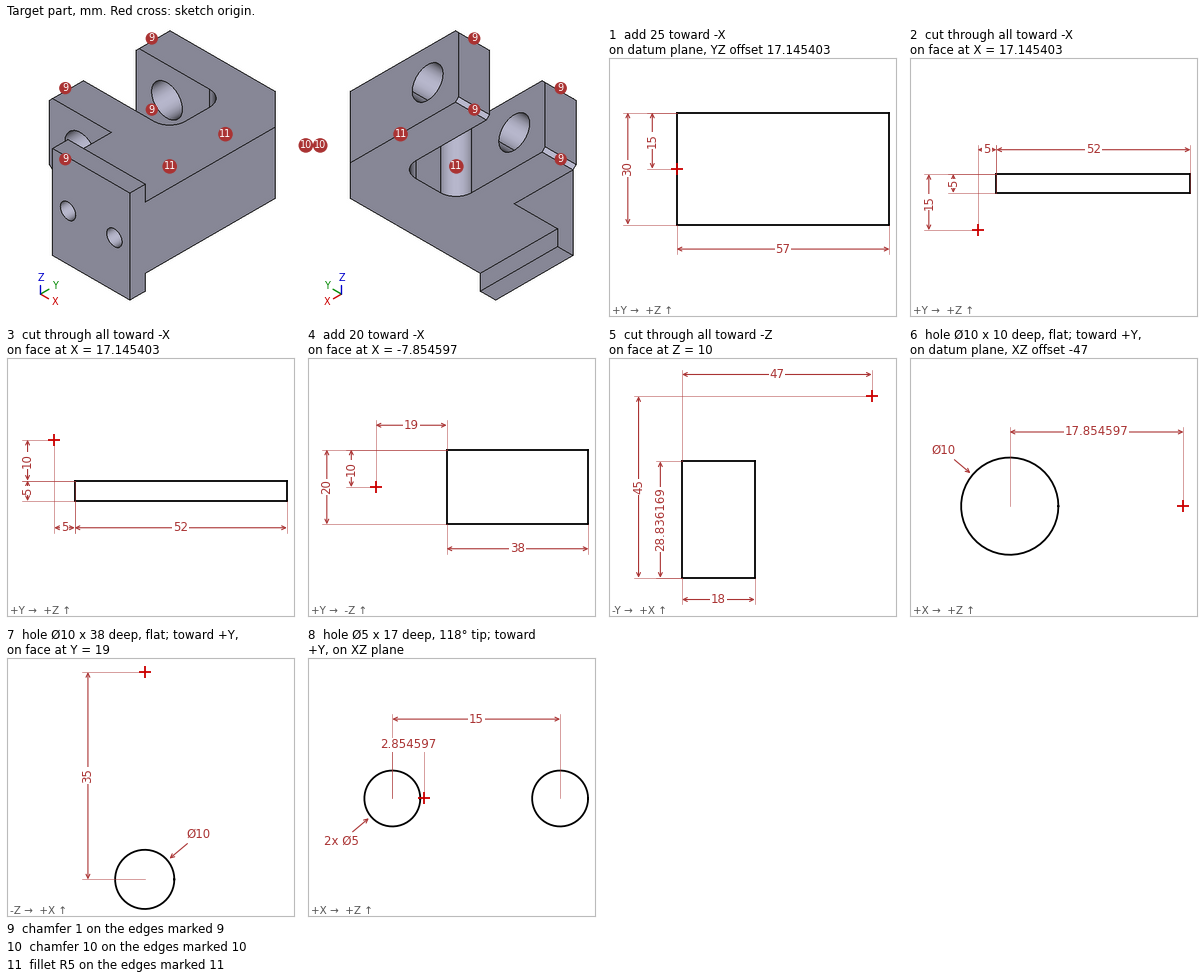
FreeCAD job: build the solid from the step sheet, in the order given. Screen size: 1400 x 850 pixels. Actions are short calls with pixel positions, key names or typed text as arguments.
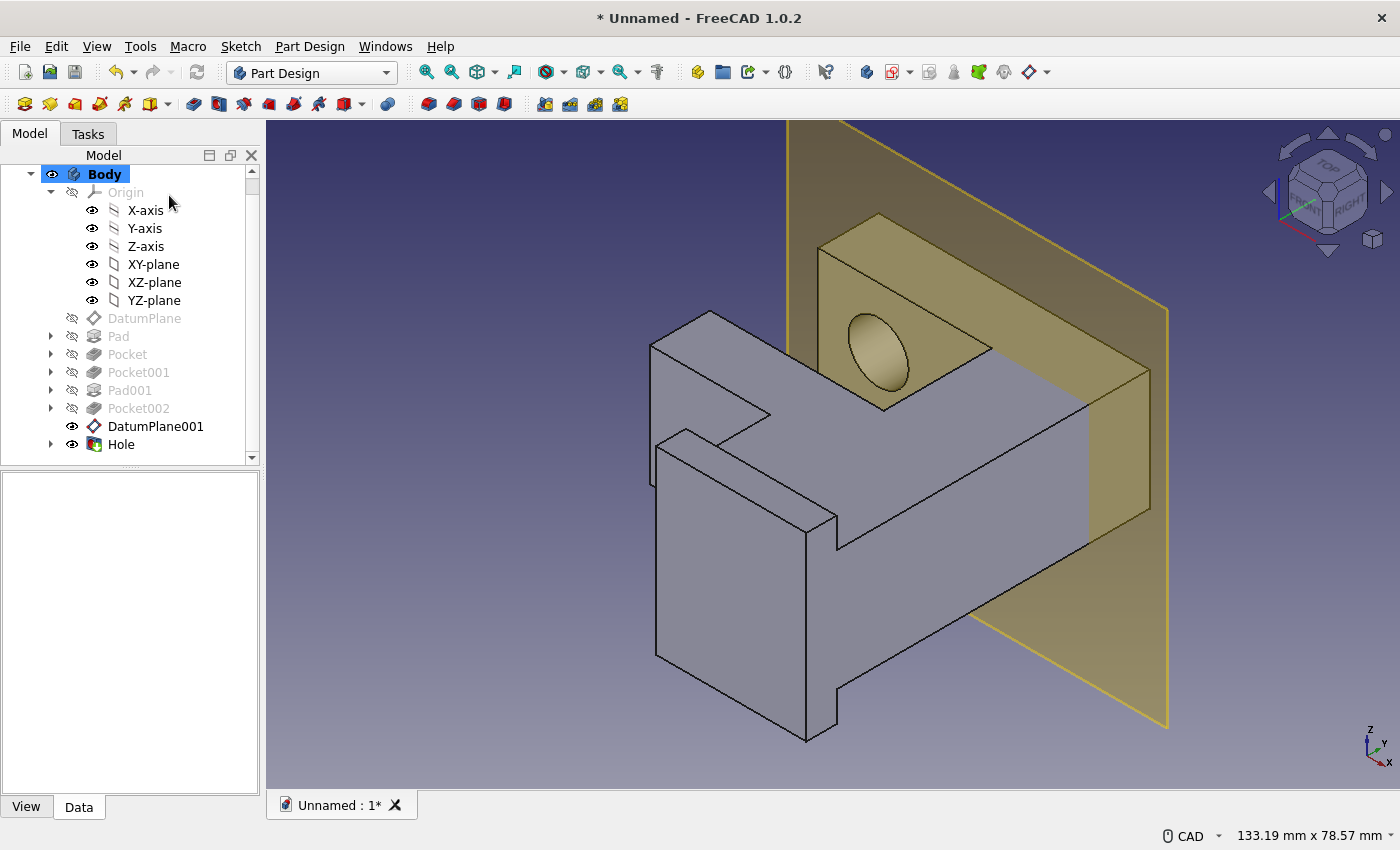
click(117, 426)
key(space)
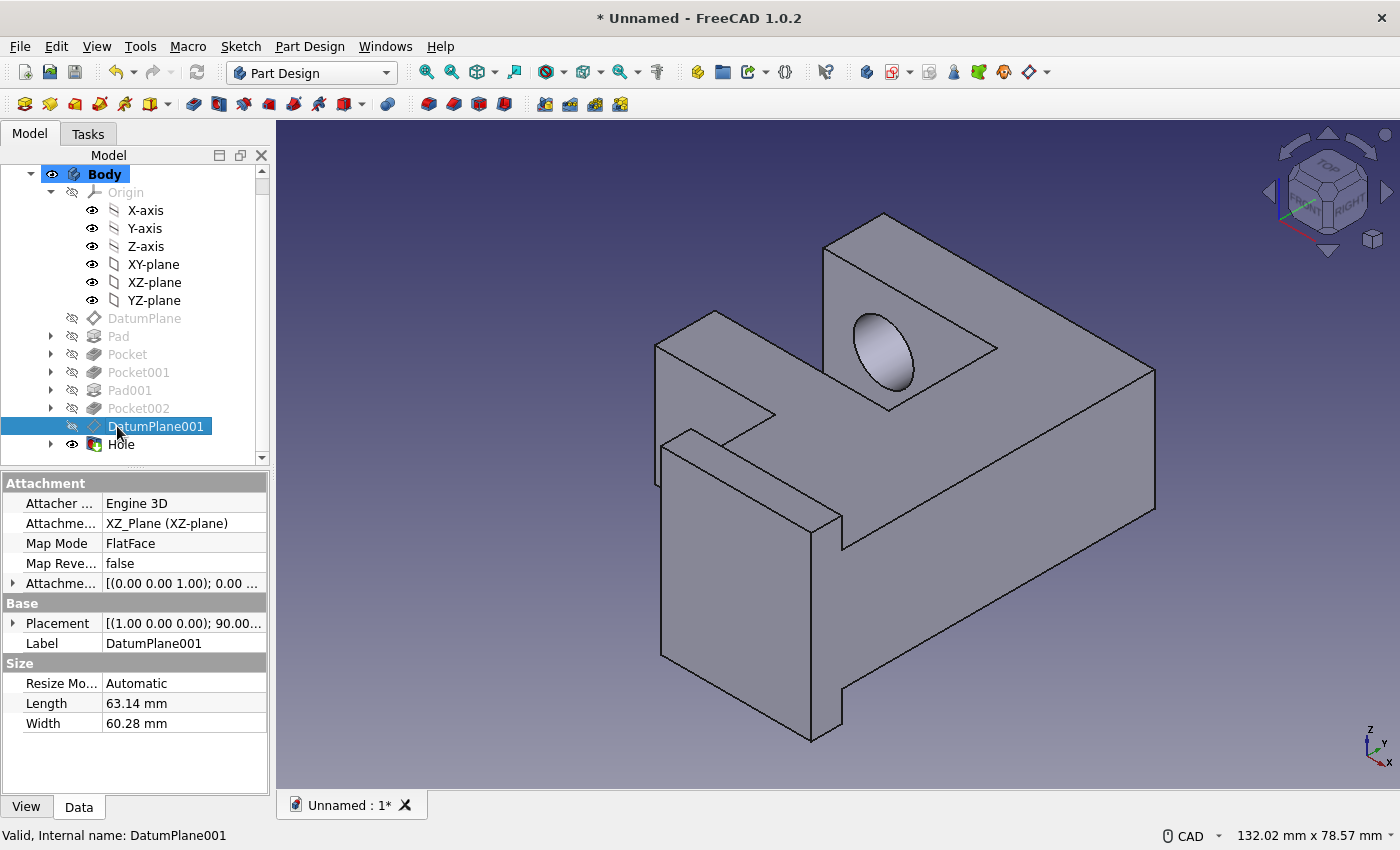
click(698, 419)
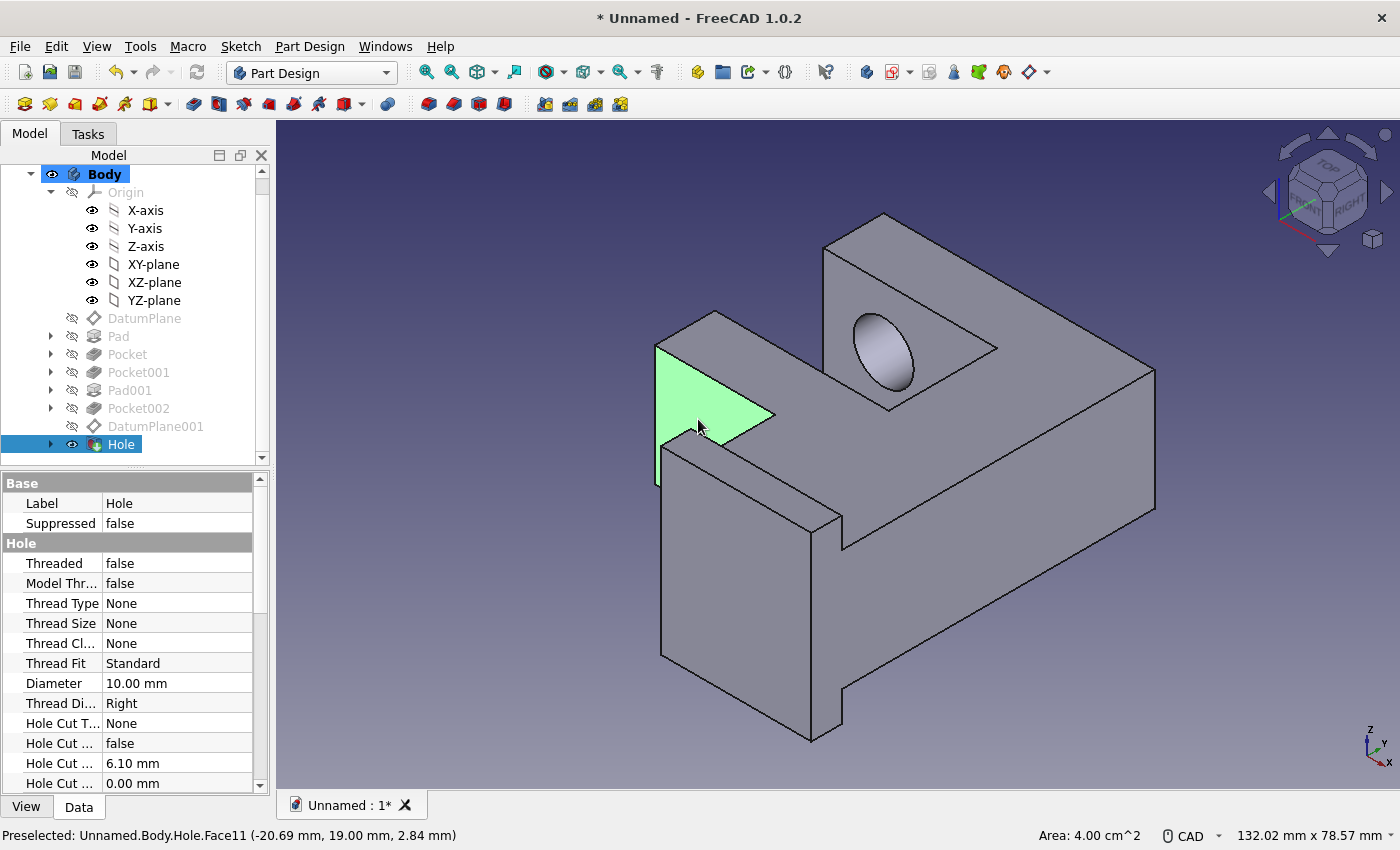
click(892, 72)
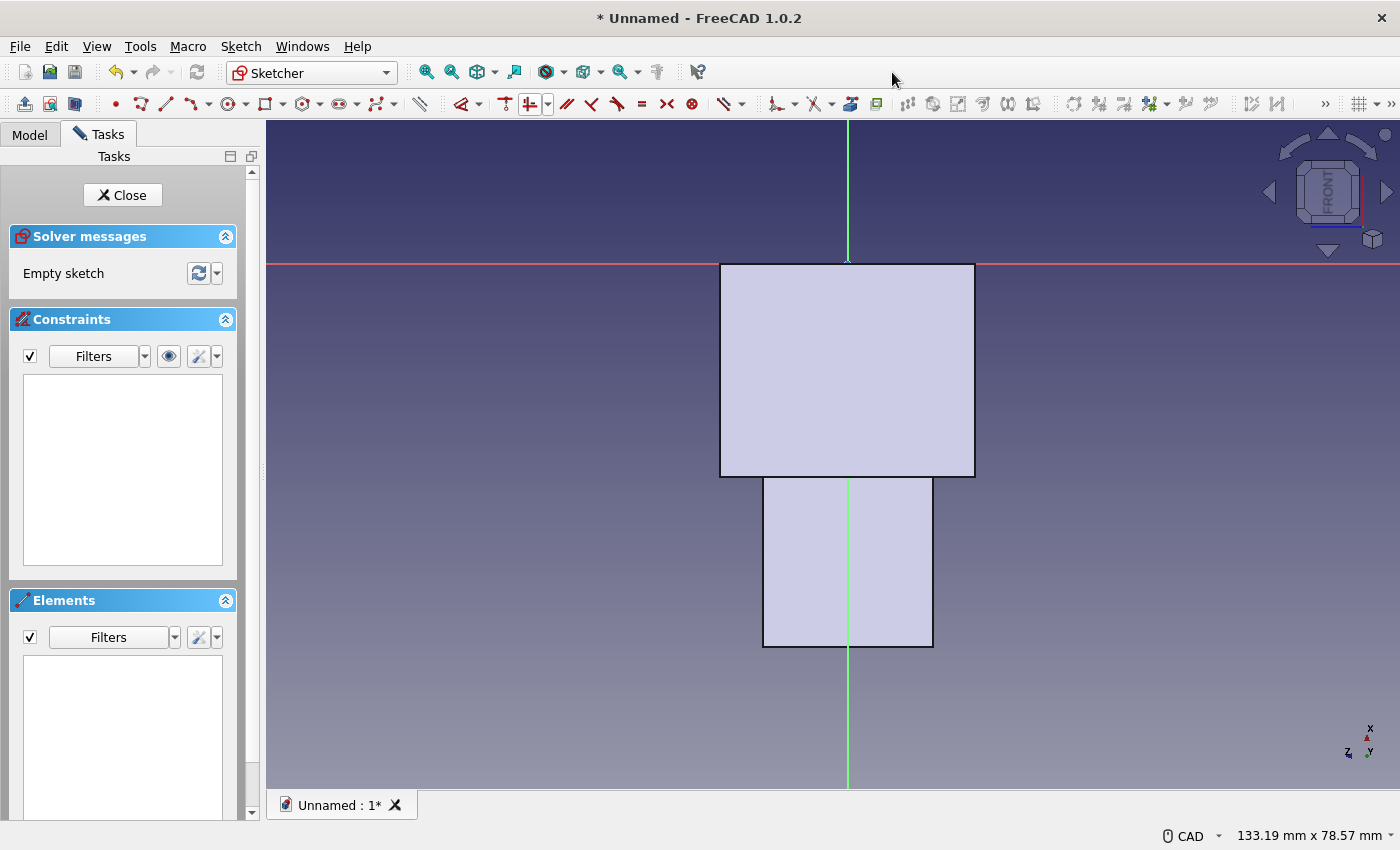
scroll(869, 589, up, 8)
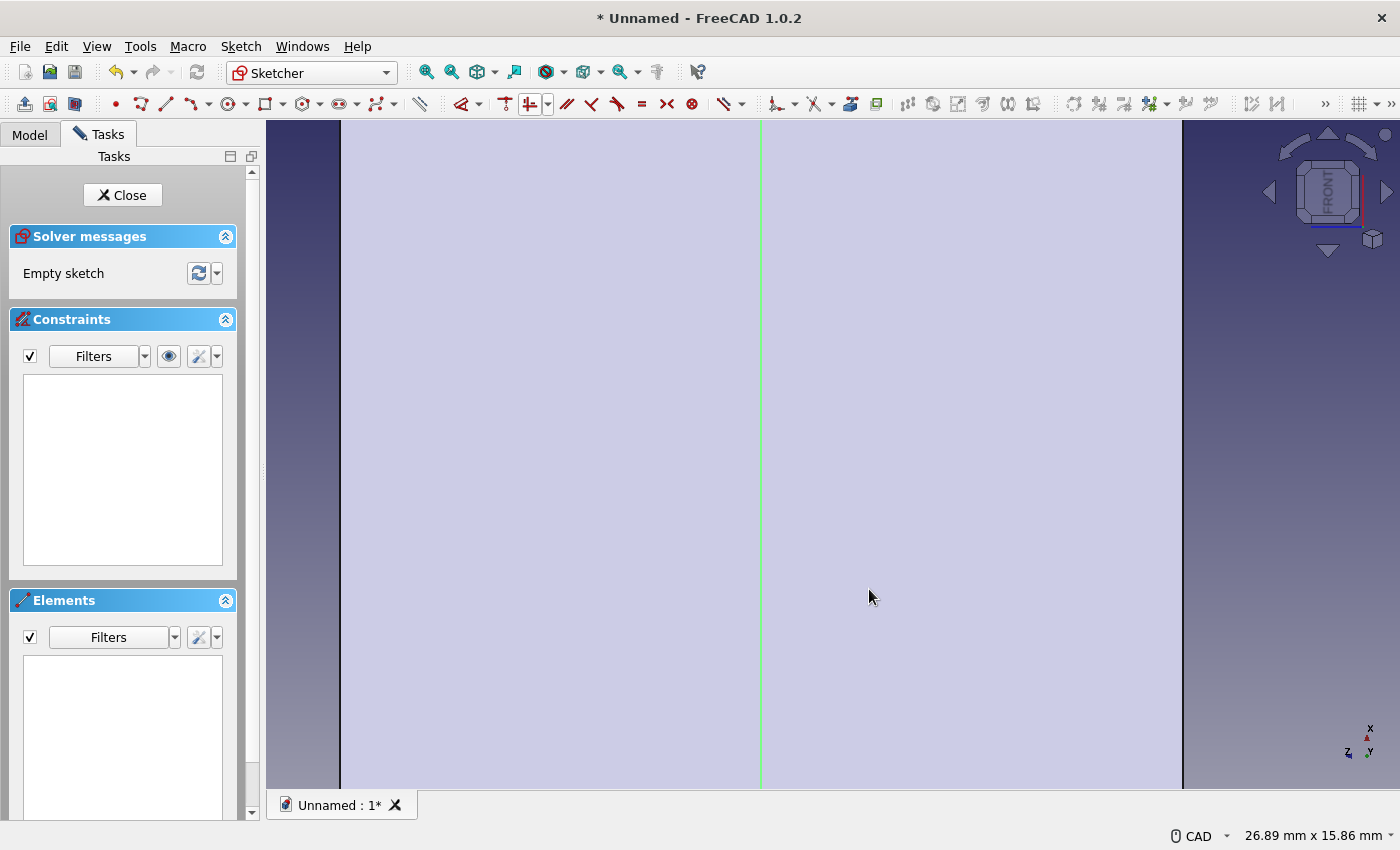
key(g)
key(c)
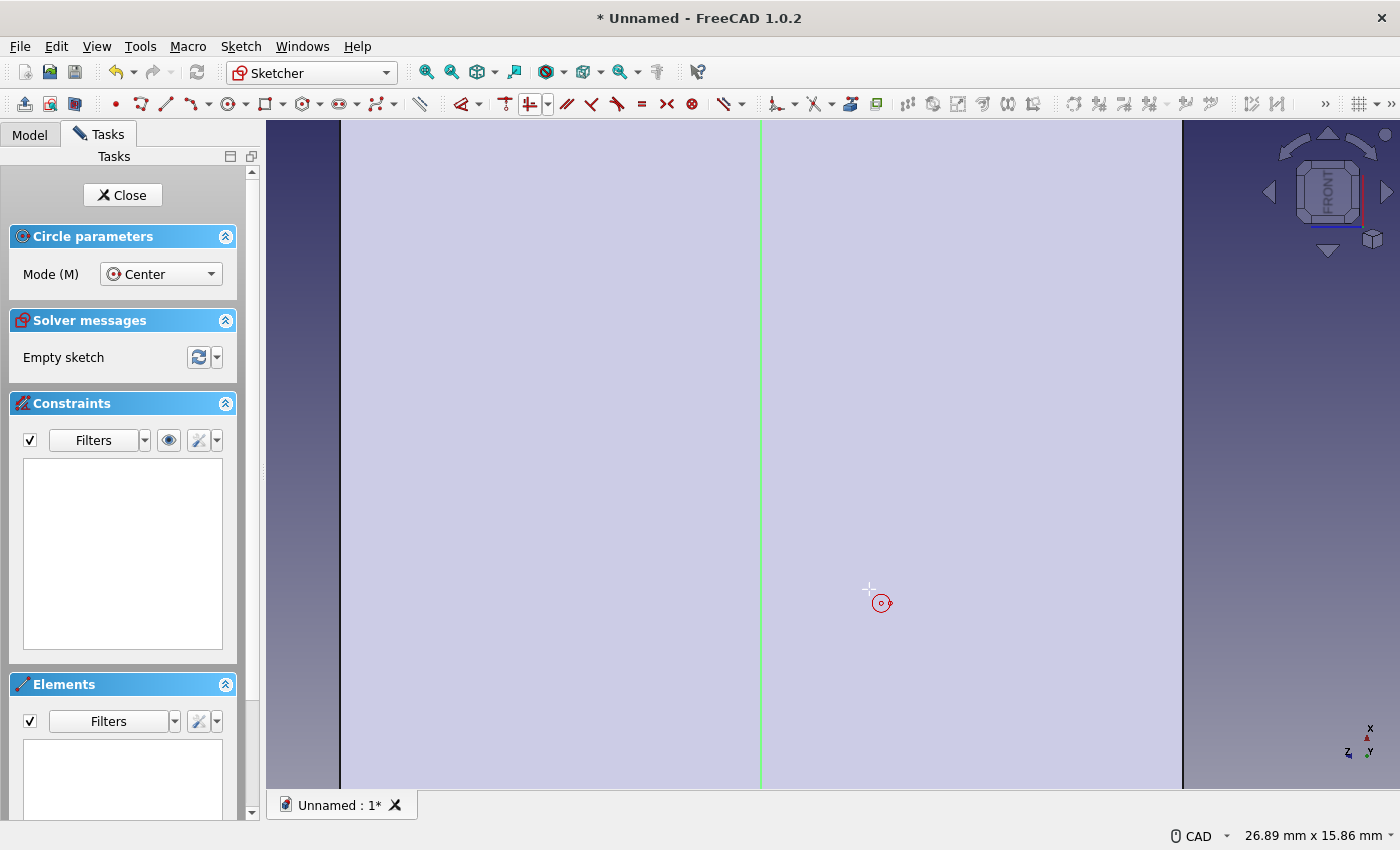
click(761, 453)
click(910, 304)
key(Escape)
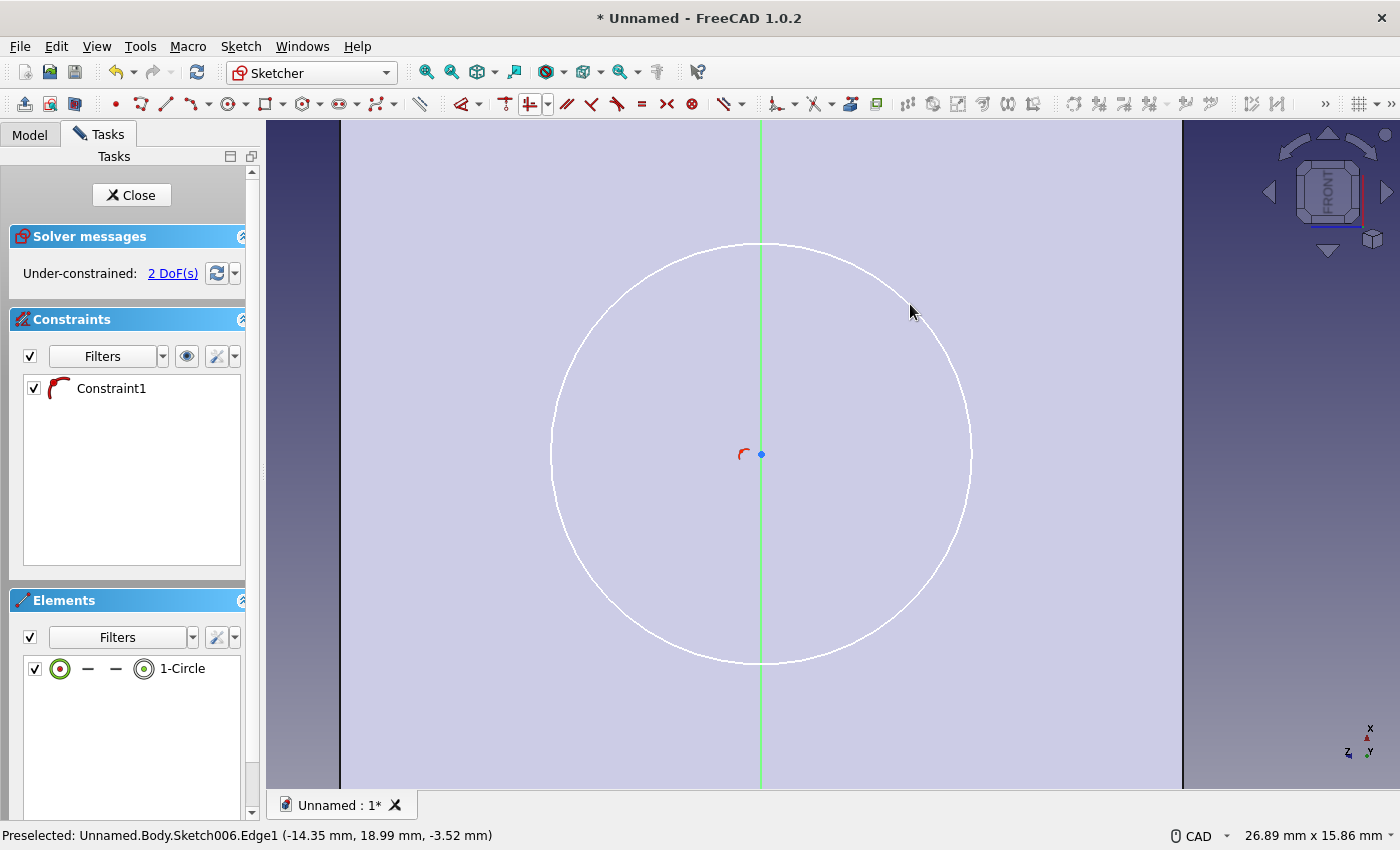
click(460, 104)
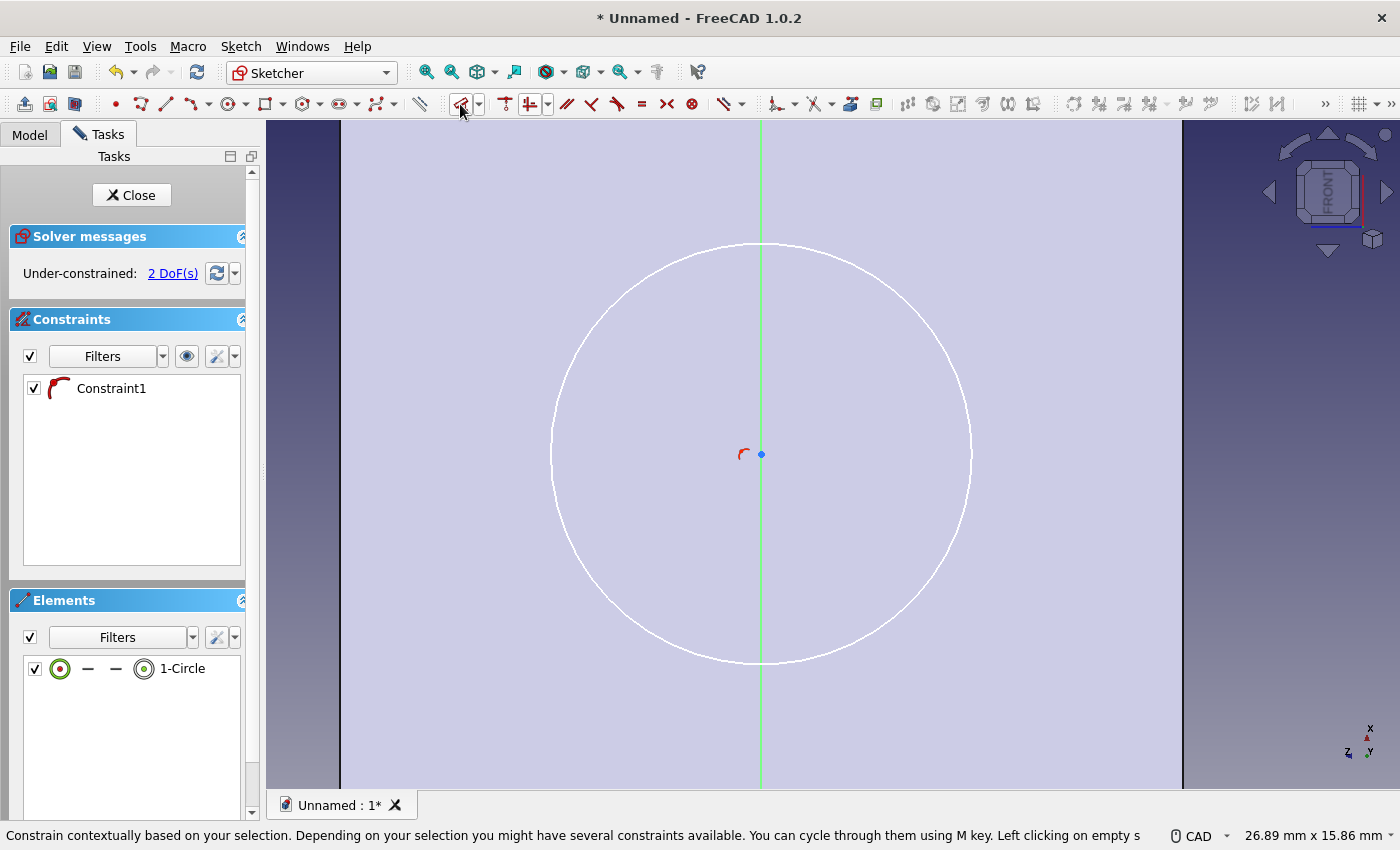
click(910, 305)
click(933, 282)